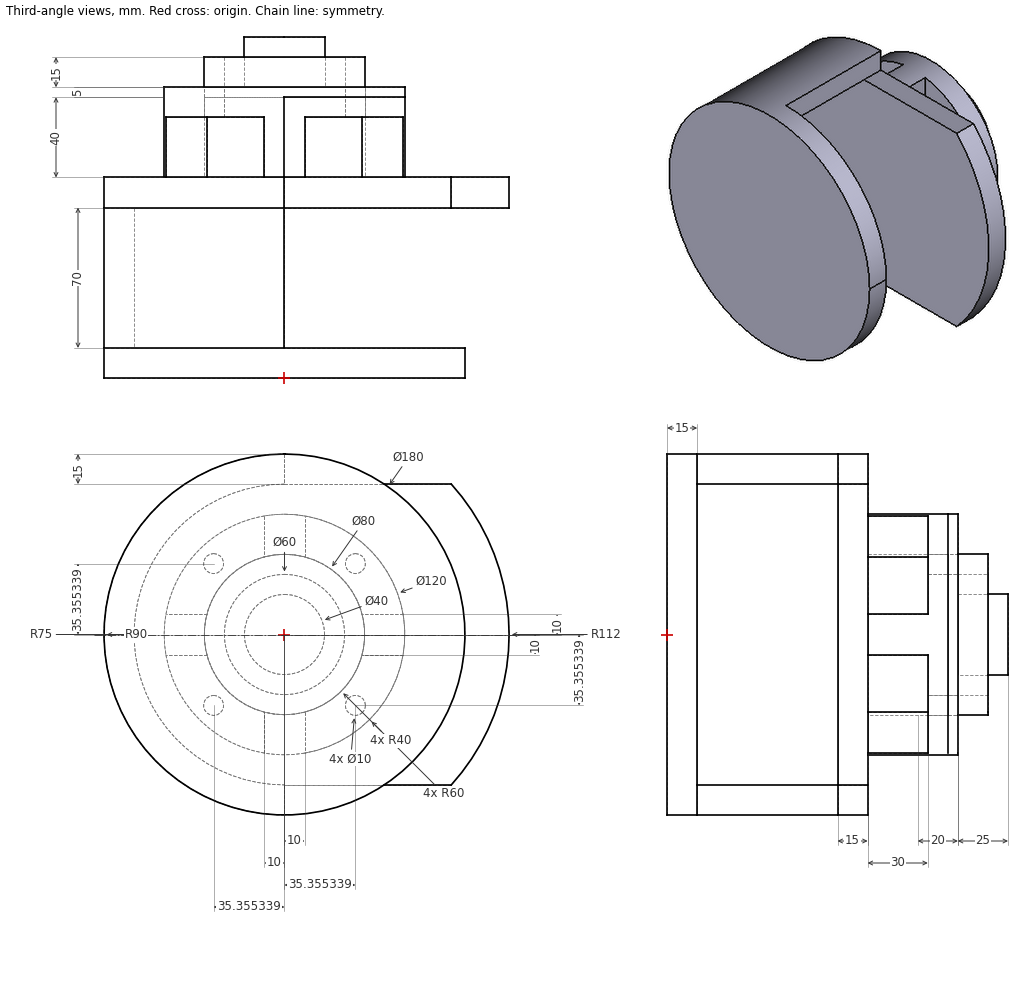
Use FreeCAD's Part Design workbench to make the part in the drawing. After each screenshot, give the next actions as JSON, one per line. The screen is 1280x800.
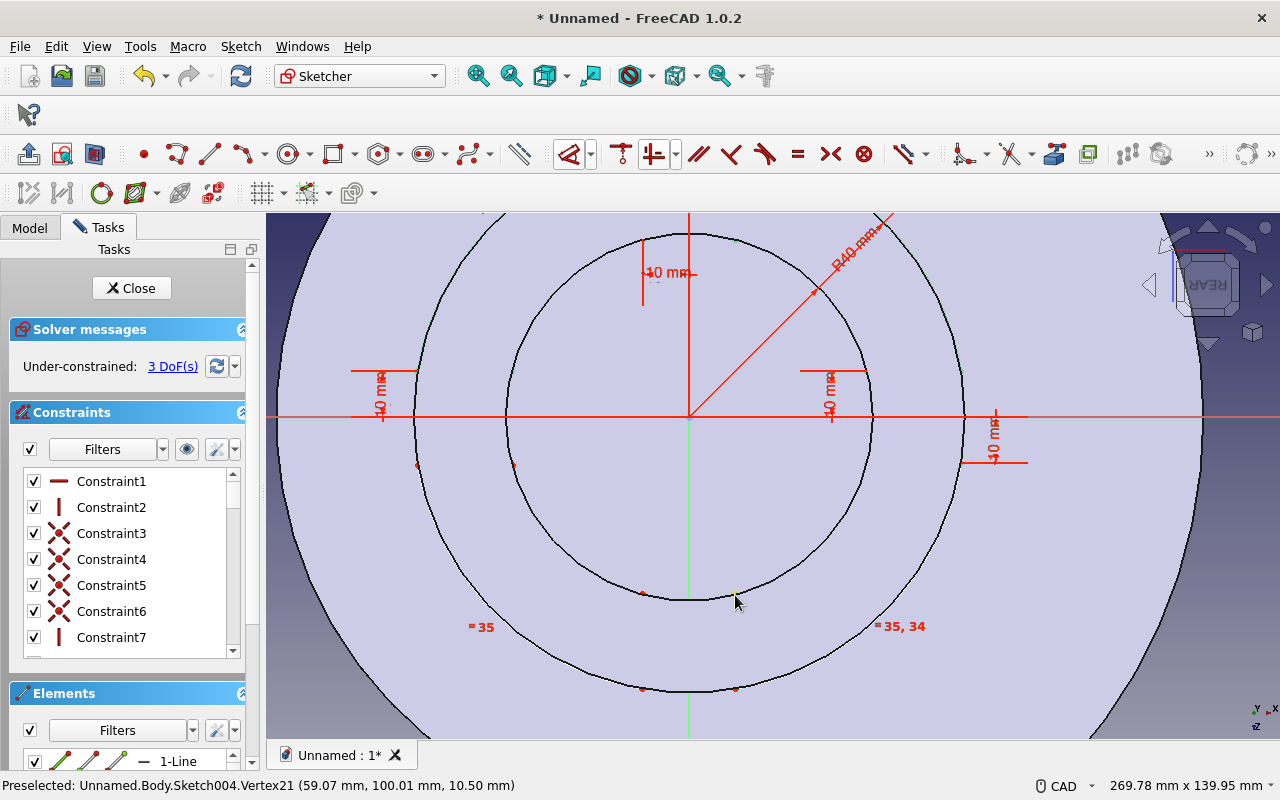
{"action": "left_click", "coordinate": [735, 595]}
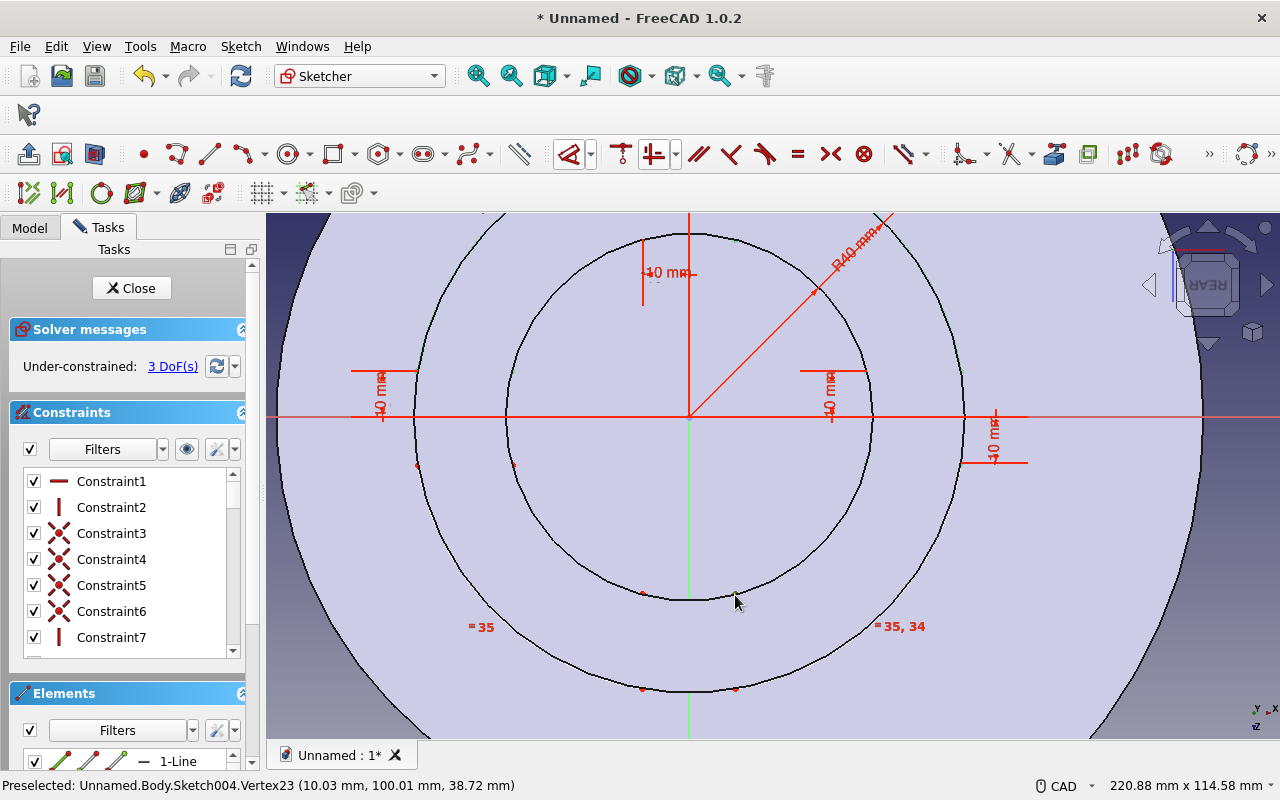
{"action": "key", "text": "l"}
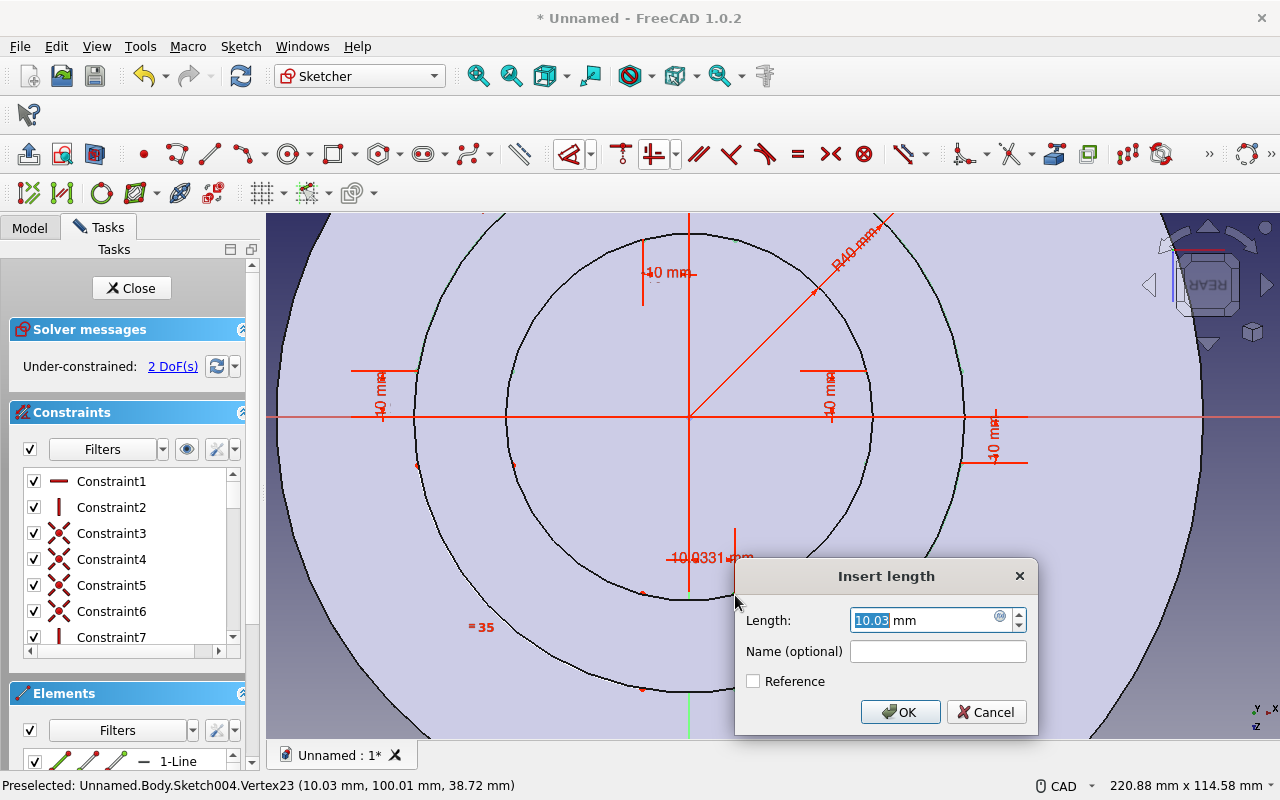
{"action": "type", "text": "10"}
{"action": "key", "text": "Return"}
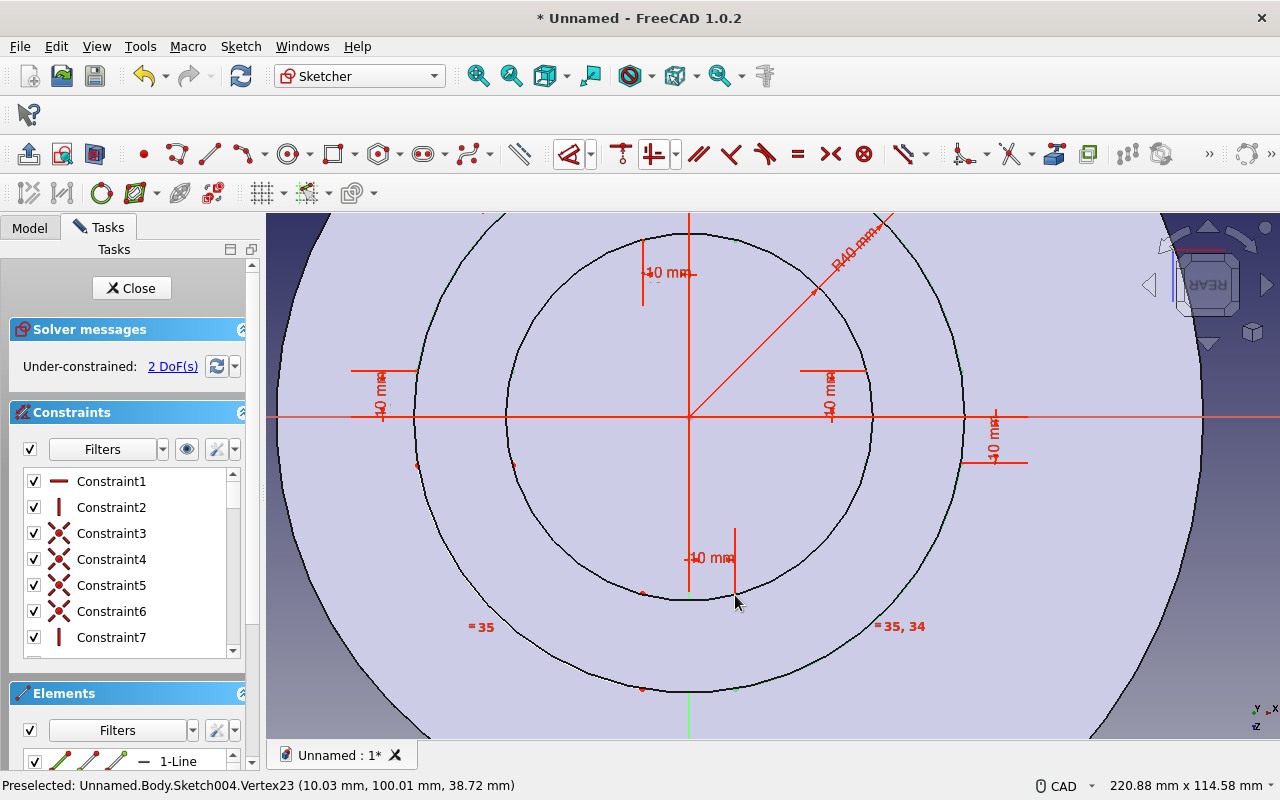
{"action": "left_click", "coordinate": [643, 689]}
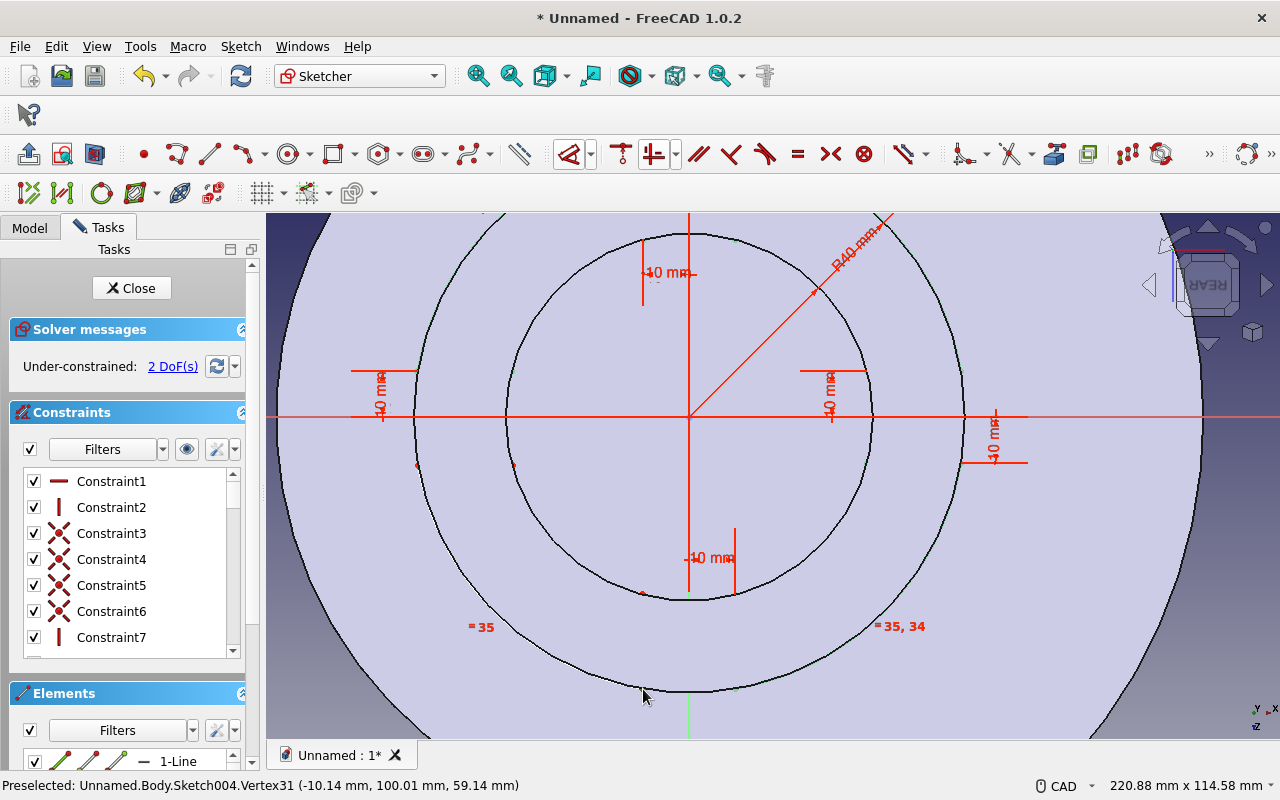
{"action": "key", "text": "l"}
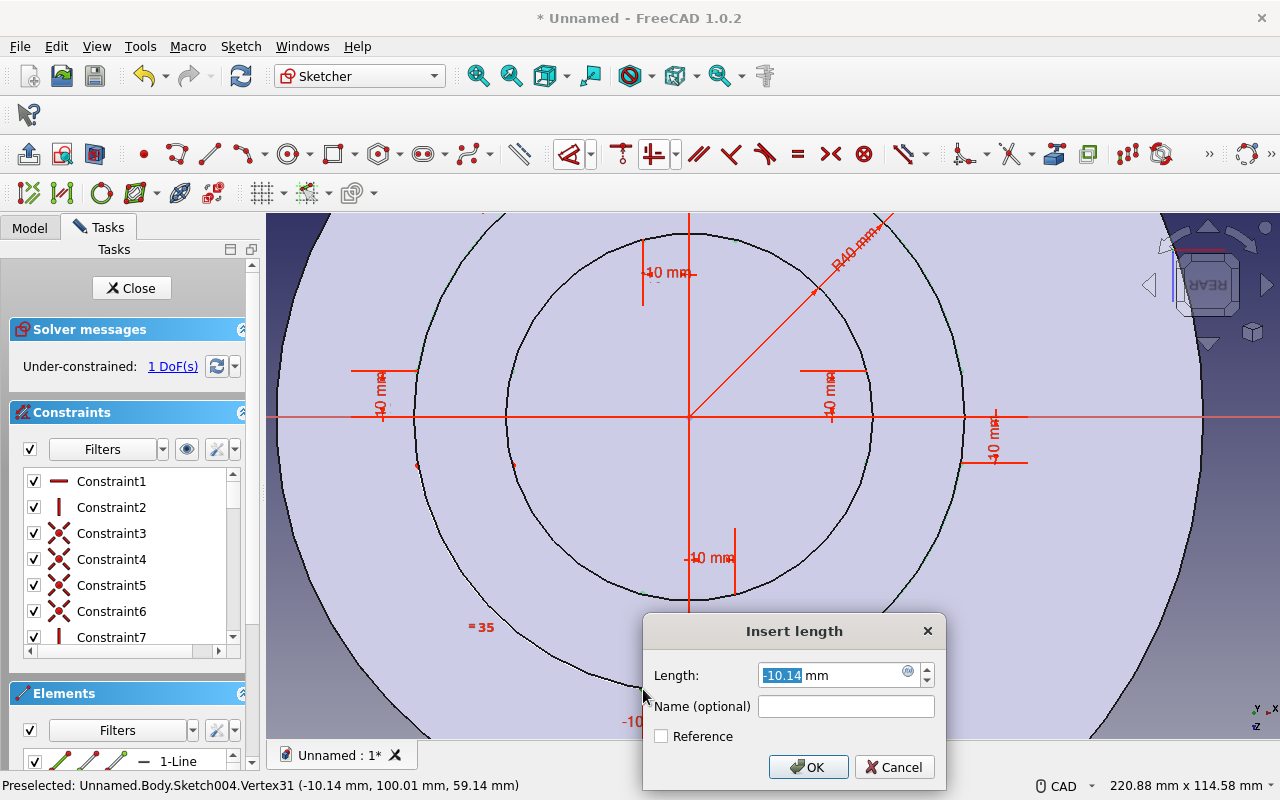
{"action": "type", "text": "-10"}
{"action": "key", "text": "Return"}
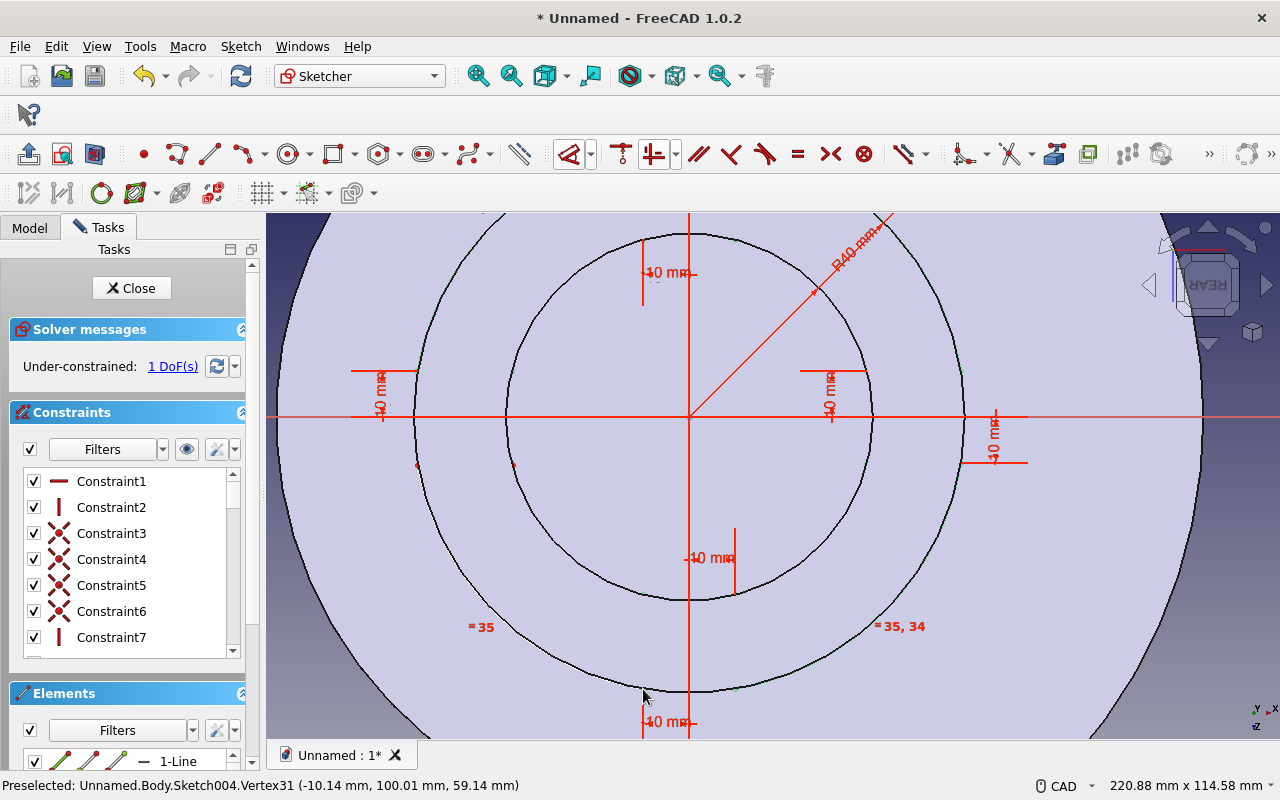
{"action": "left_click", "coordinate": [512, 465]}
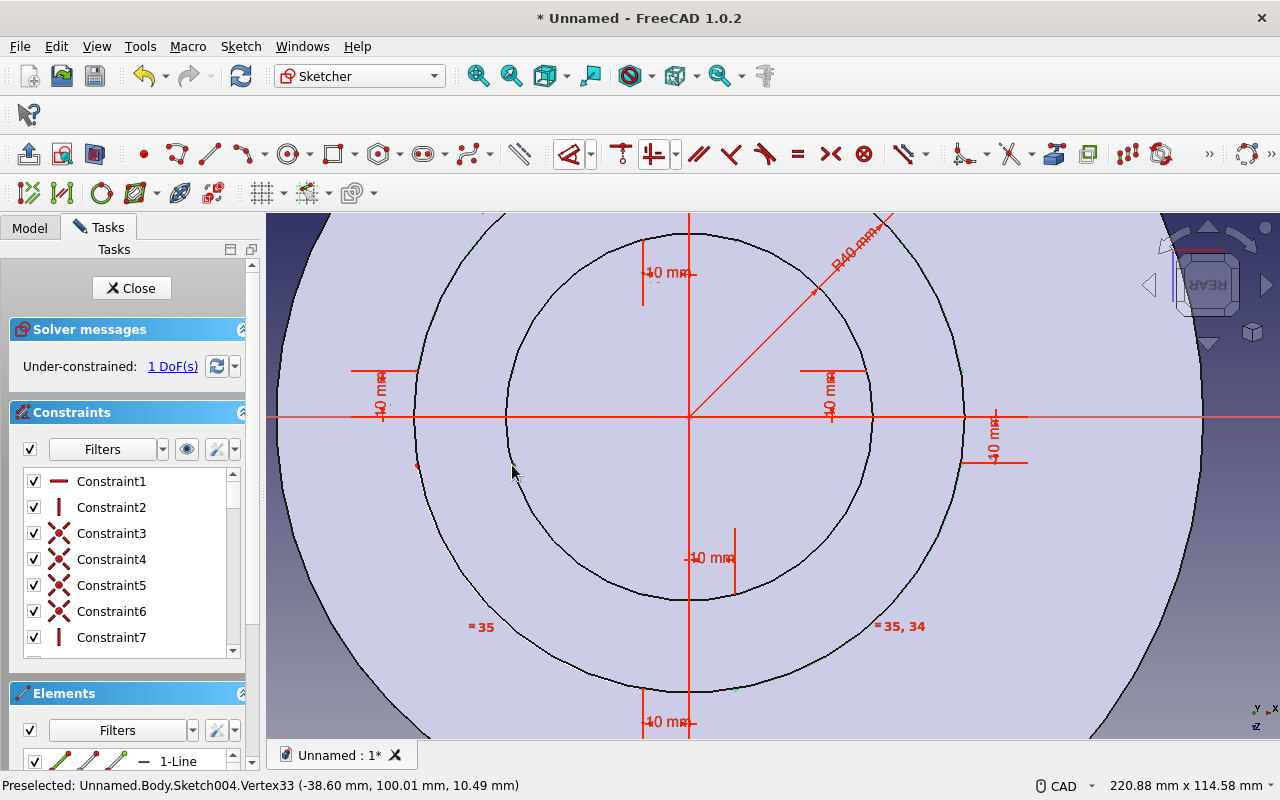
{"action": "key", "text": "i"}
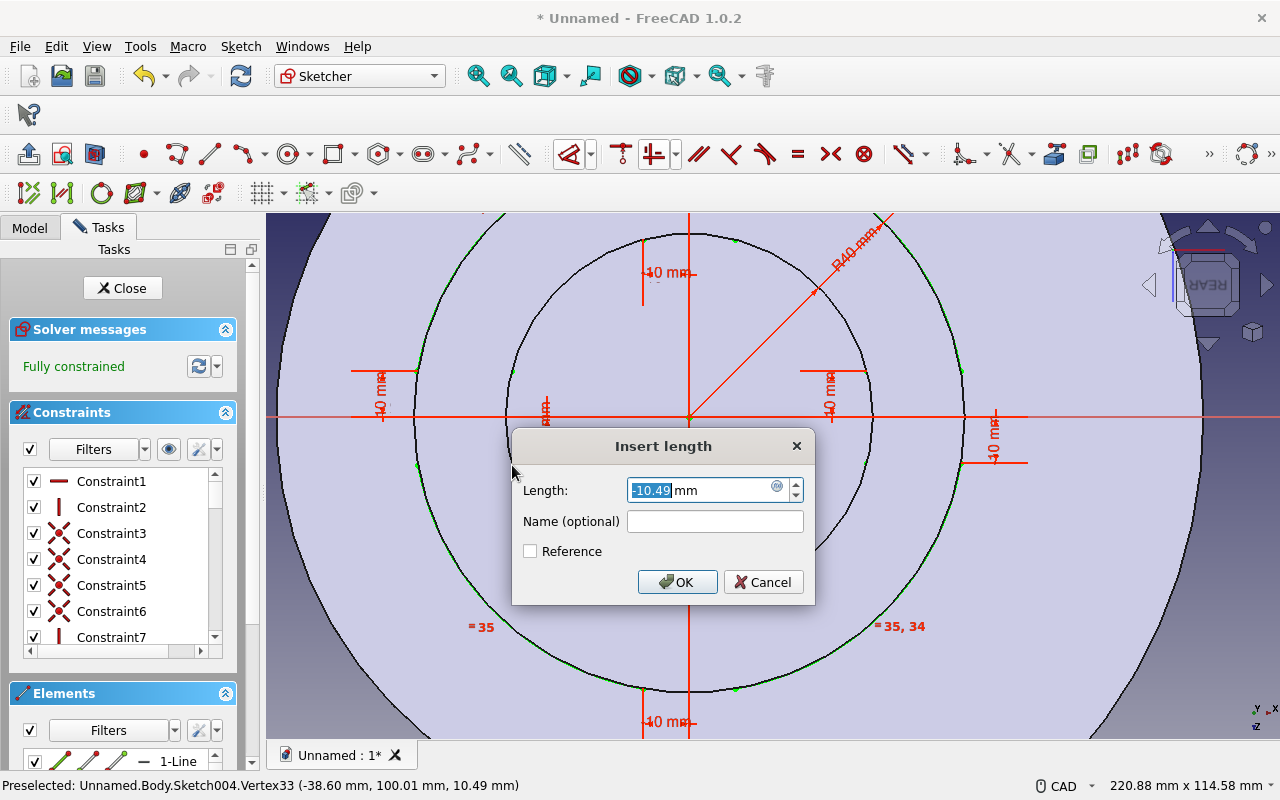
{"action": "type", "text": "-10"}
{"action": "key", "text": "Return"}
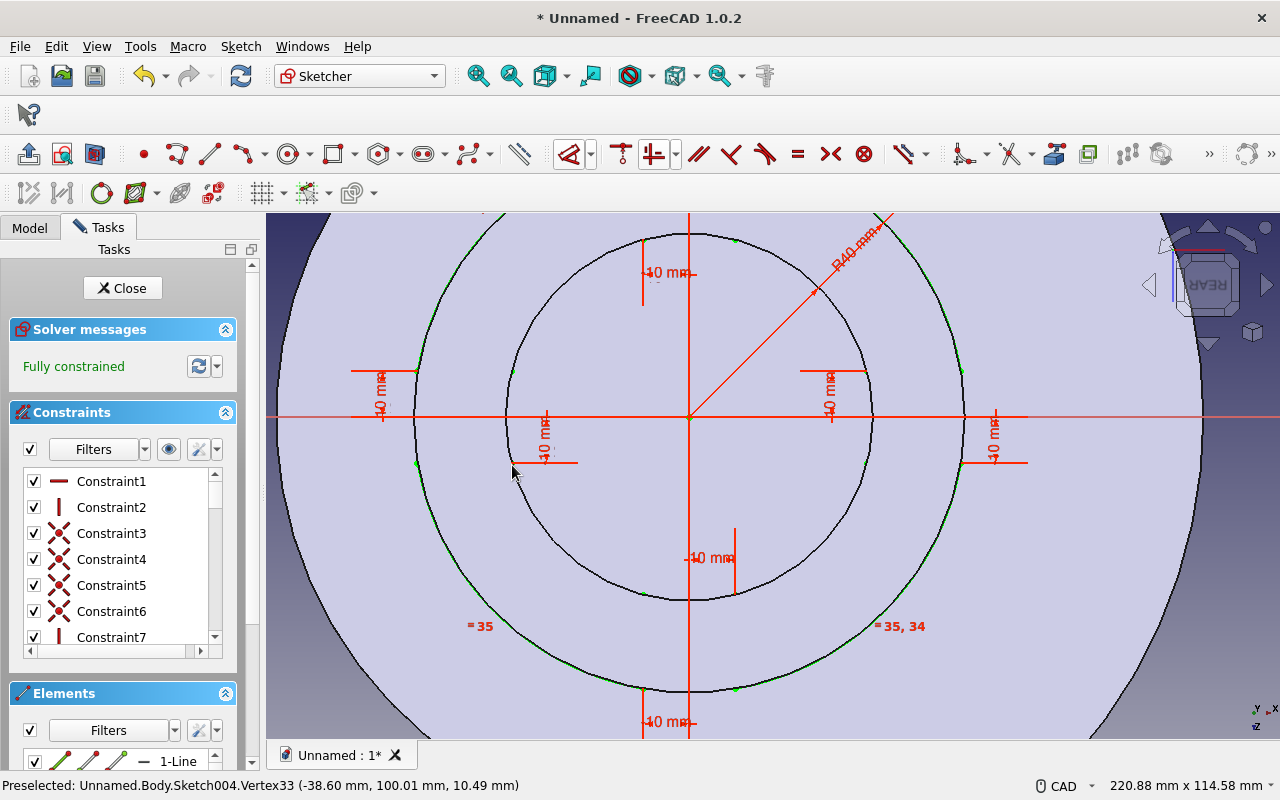
{"action": "left_click", "coordinate": [123, 288]}